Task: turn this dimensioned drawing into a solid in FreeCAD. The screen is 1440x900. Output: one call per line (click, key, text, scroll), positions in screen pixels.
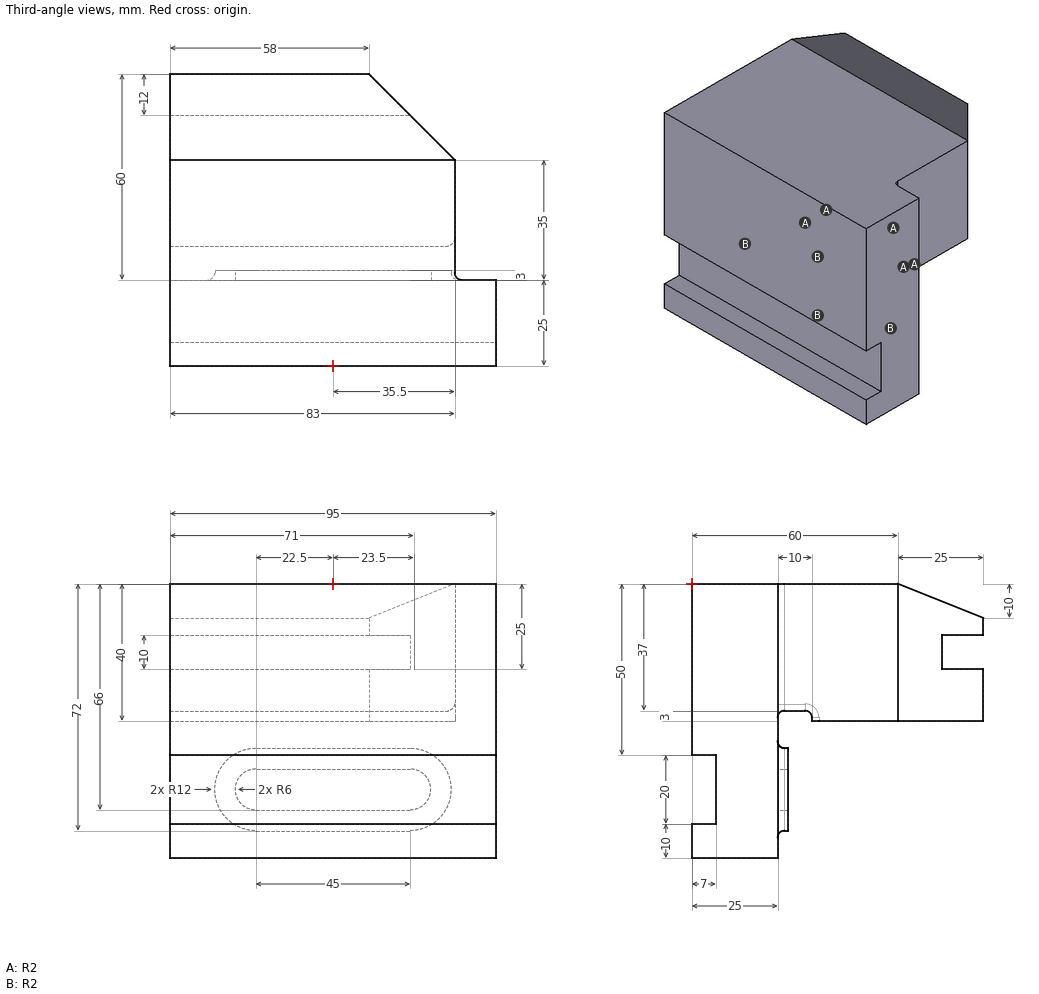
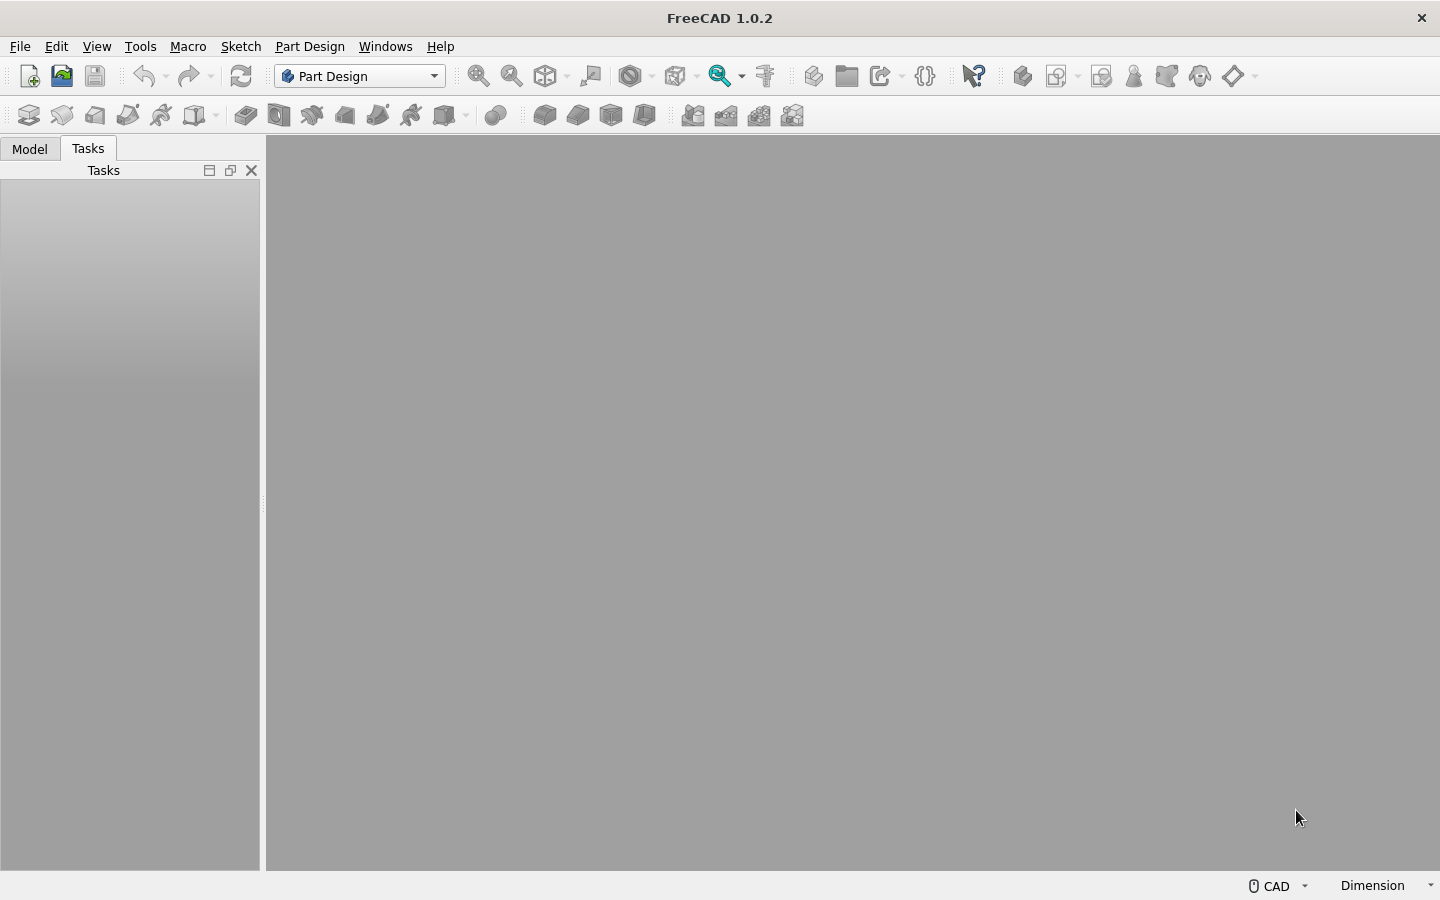
click(29, 76)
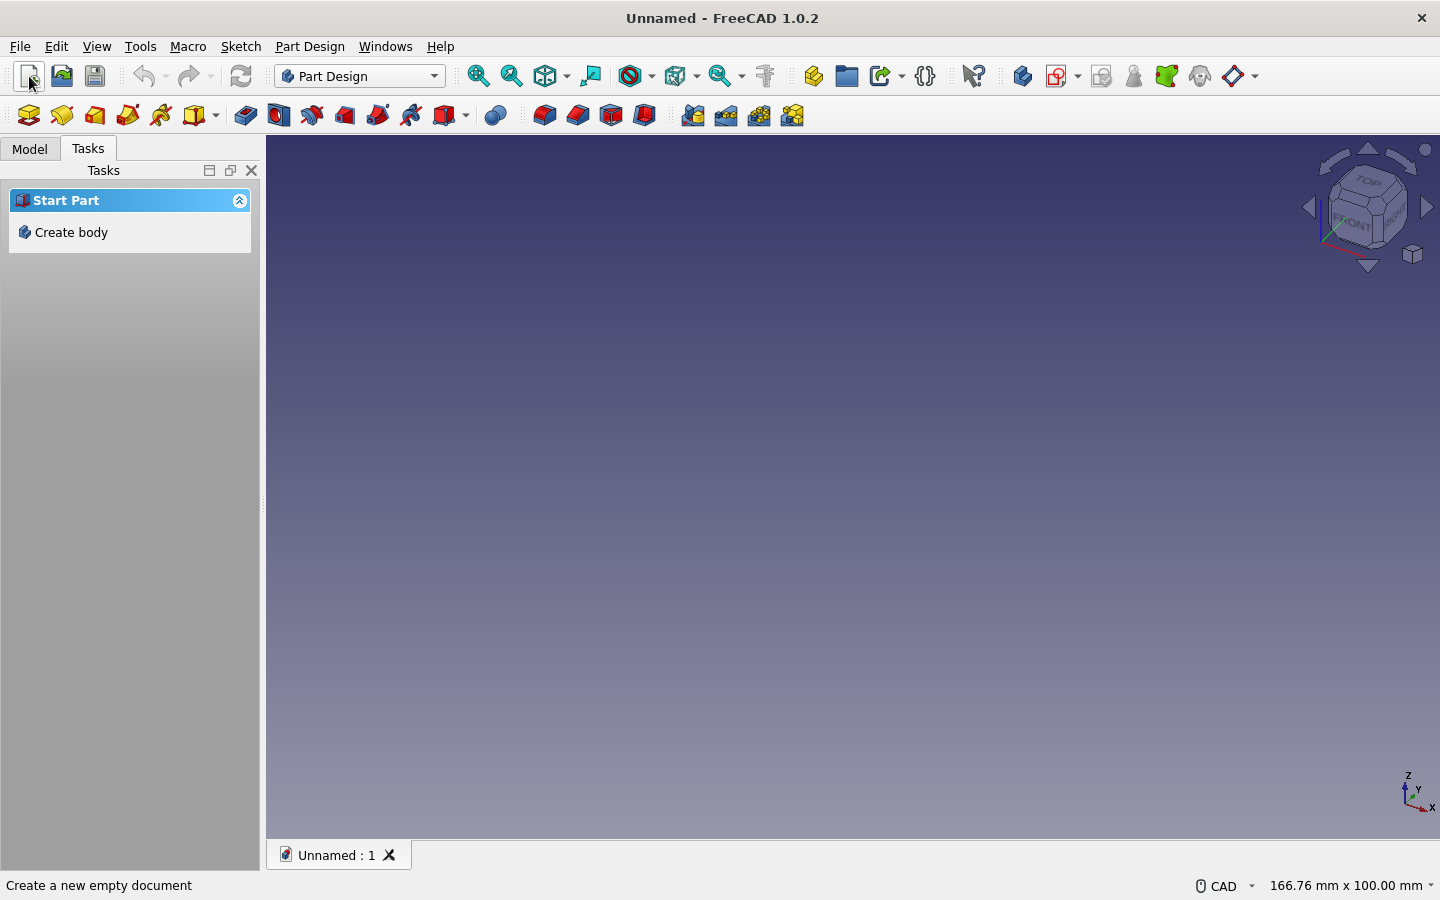
click(1056, 76)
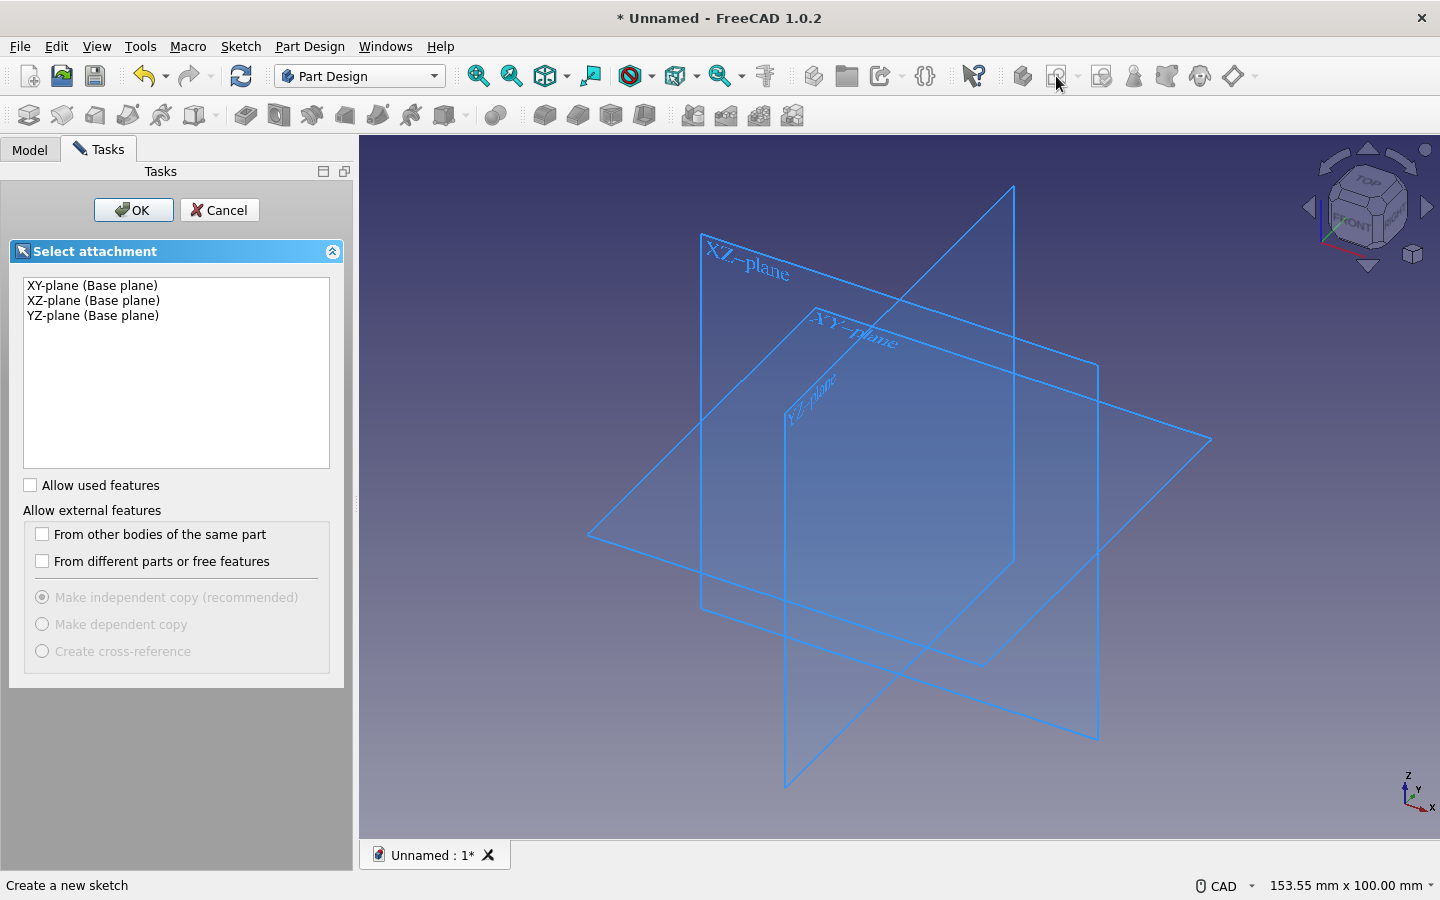
click(84, 316)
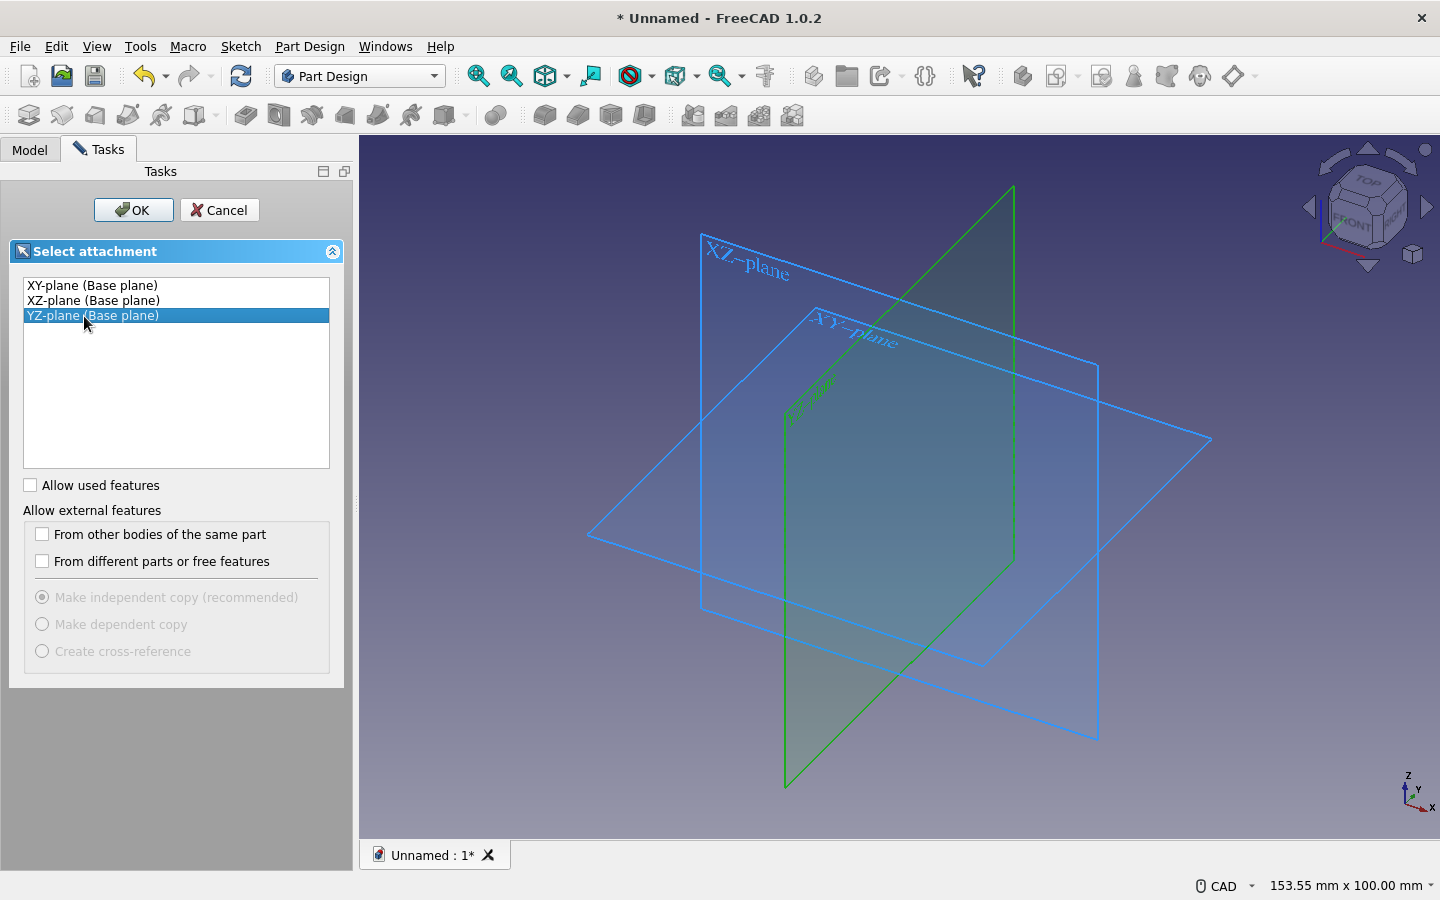
click(134, 210)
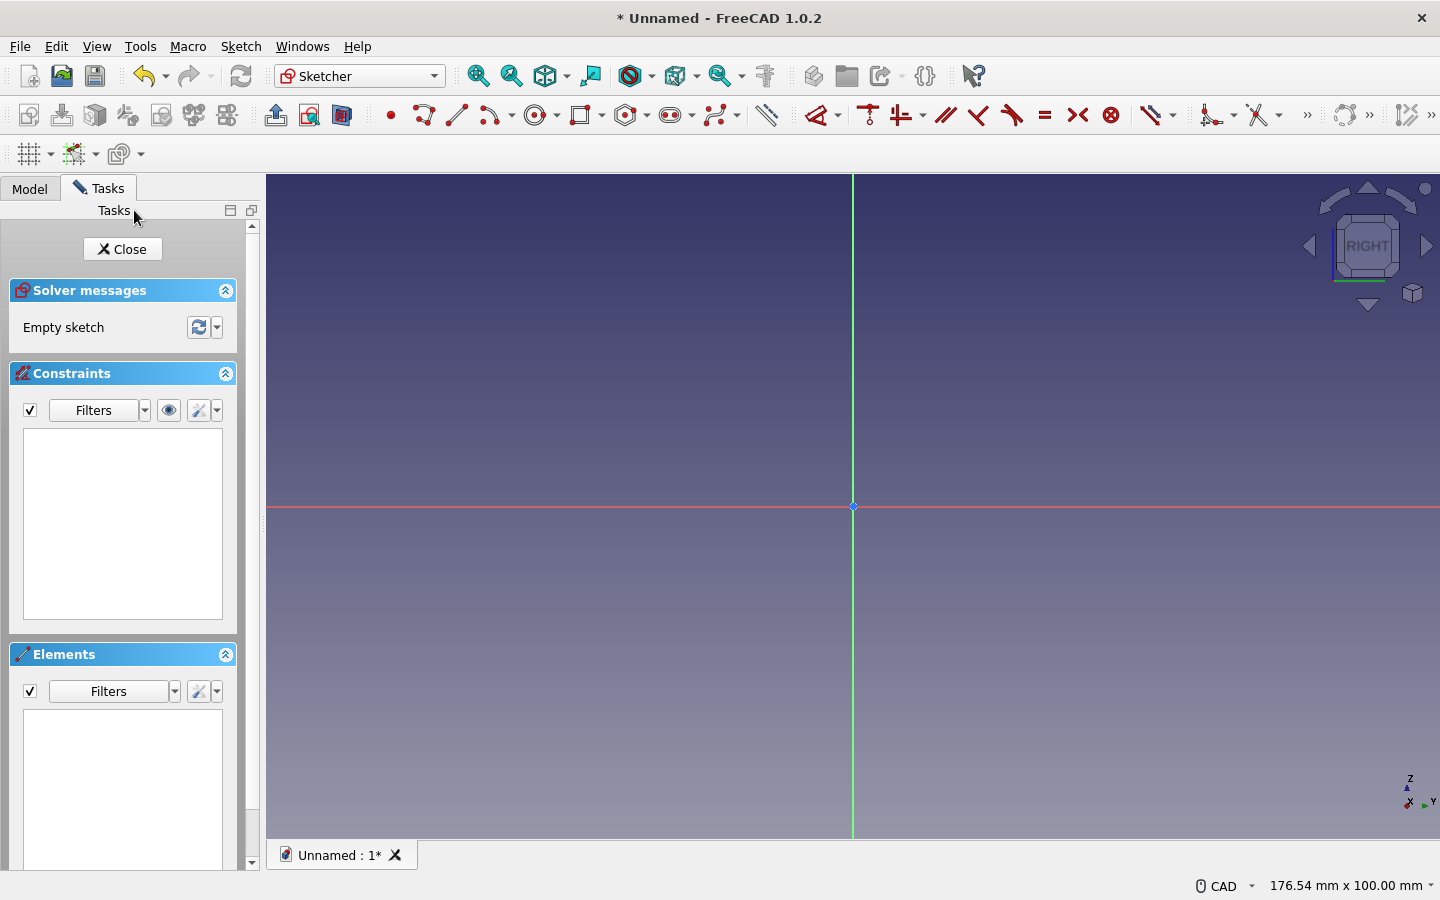
scroll(476, 202, down, 2)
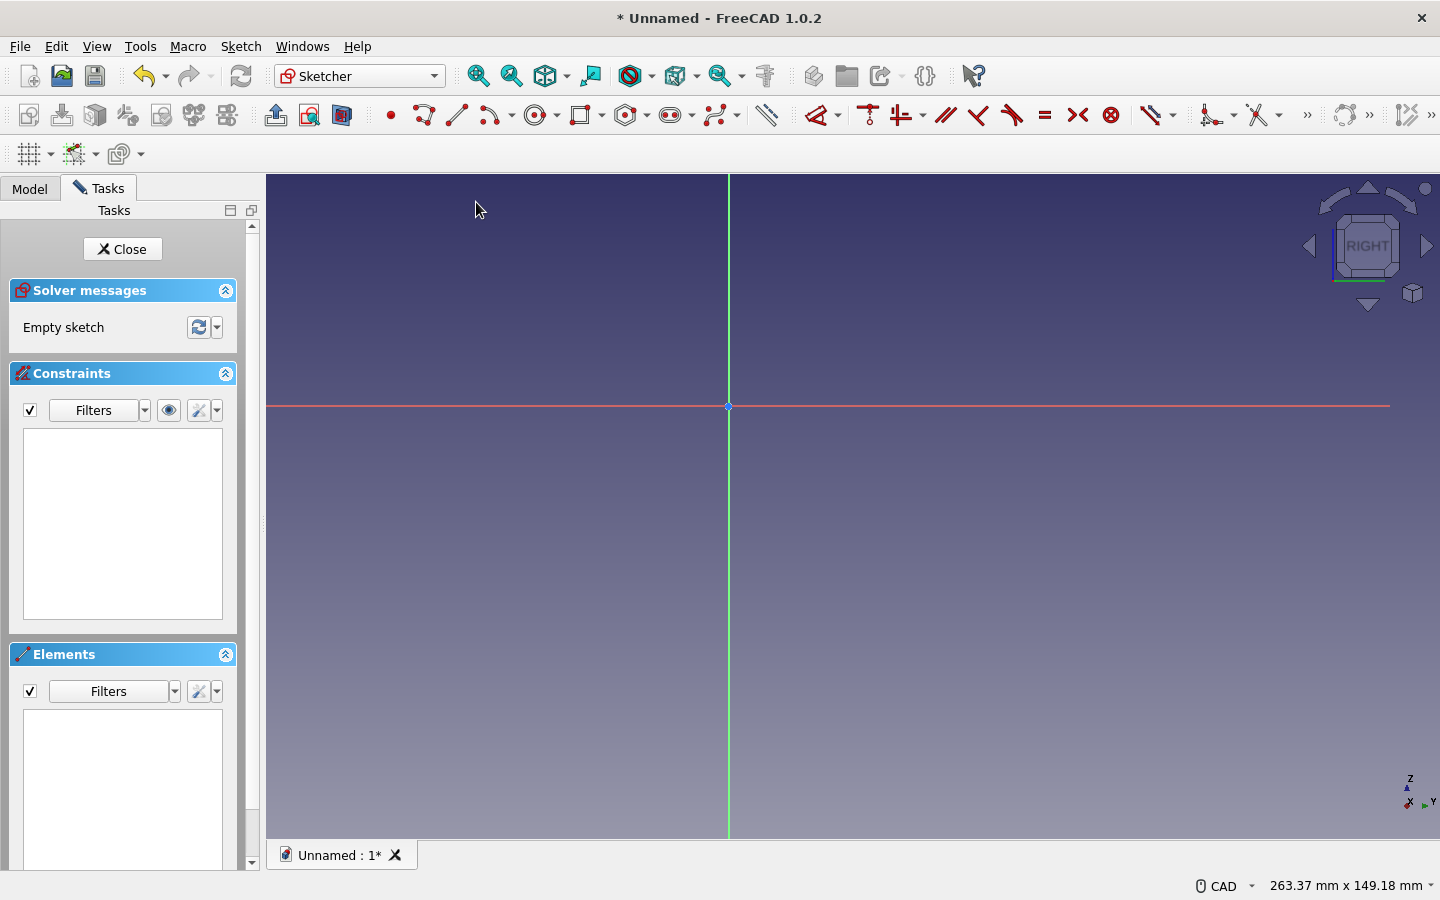
click(424, 116)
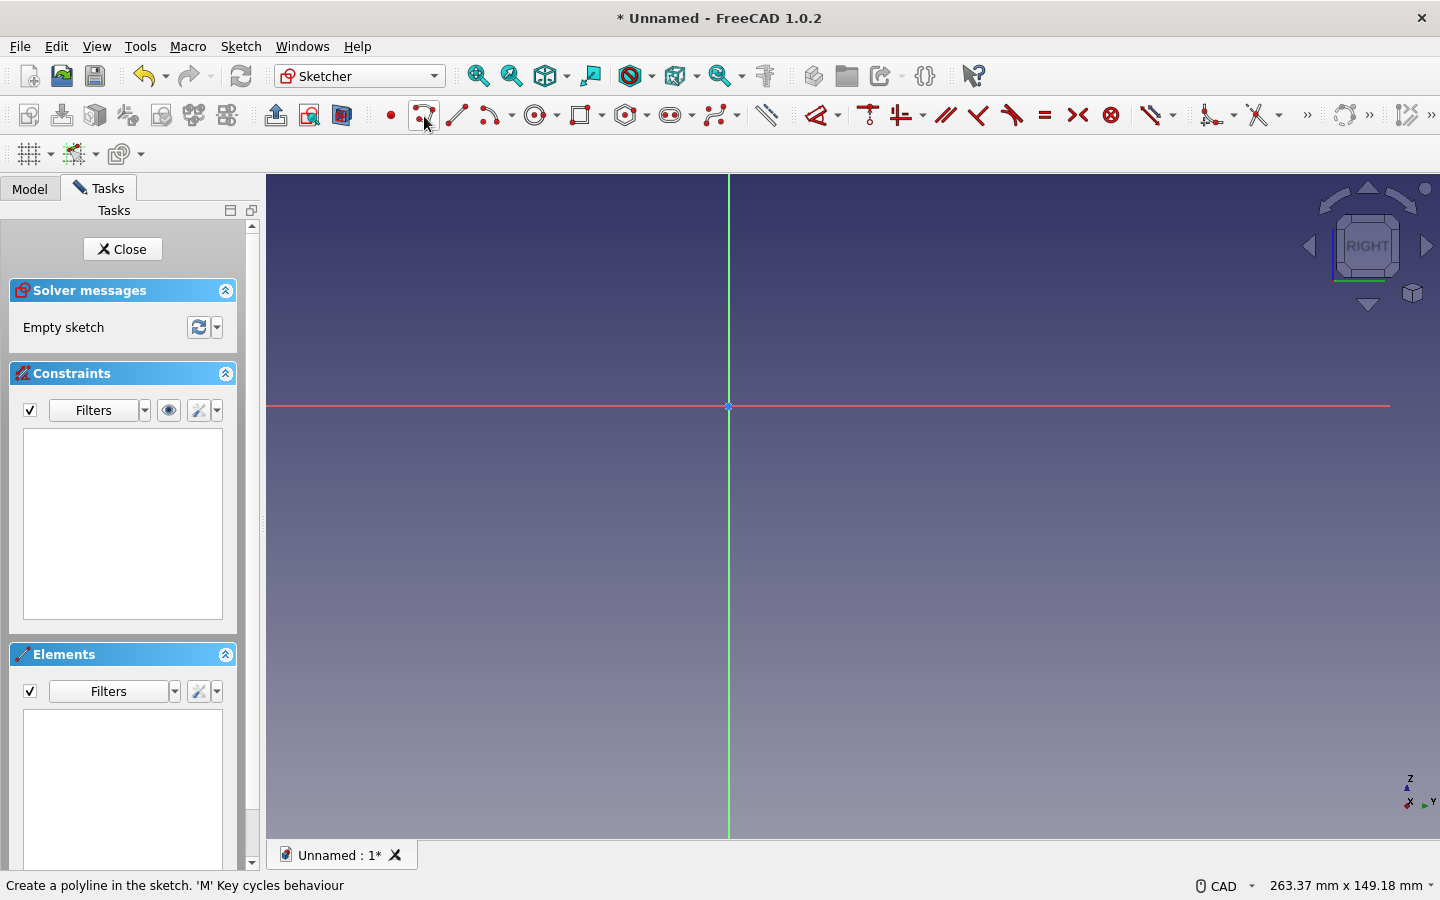
click(729, 406)
click(738, 629)
click(760, 629)
click(760, 718)
click(729, 718)
click(738, 763)
click(840, 763)
click(840, 415)
click(729, 406)
key(Escape)
key(Escape)